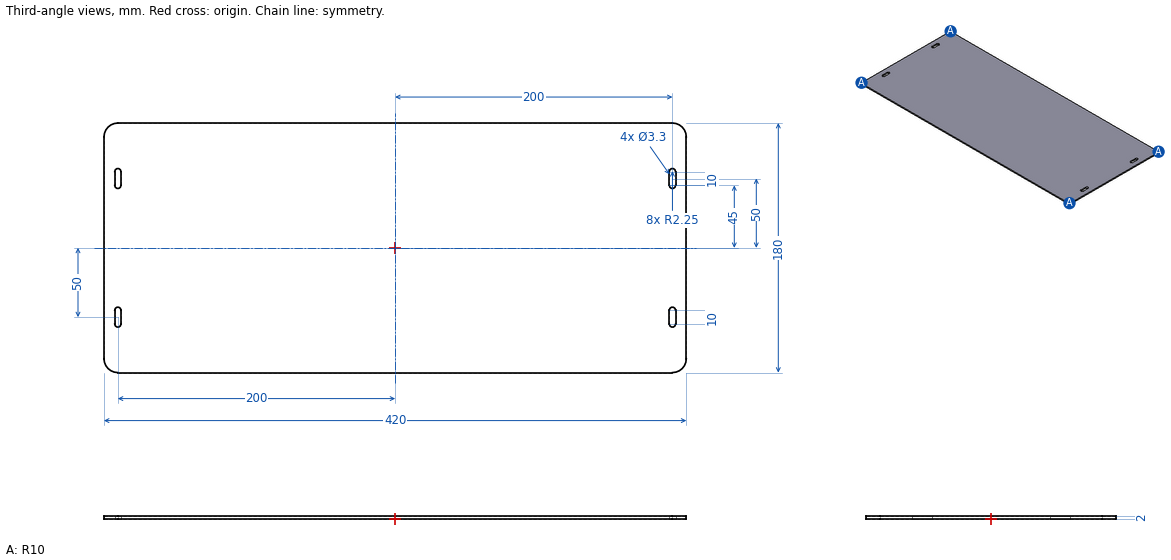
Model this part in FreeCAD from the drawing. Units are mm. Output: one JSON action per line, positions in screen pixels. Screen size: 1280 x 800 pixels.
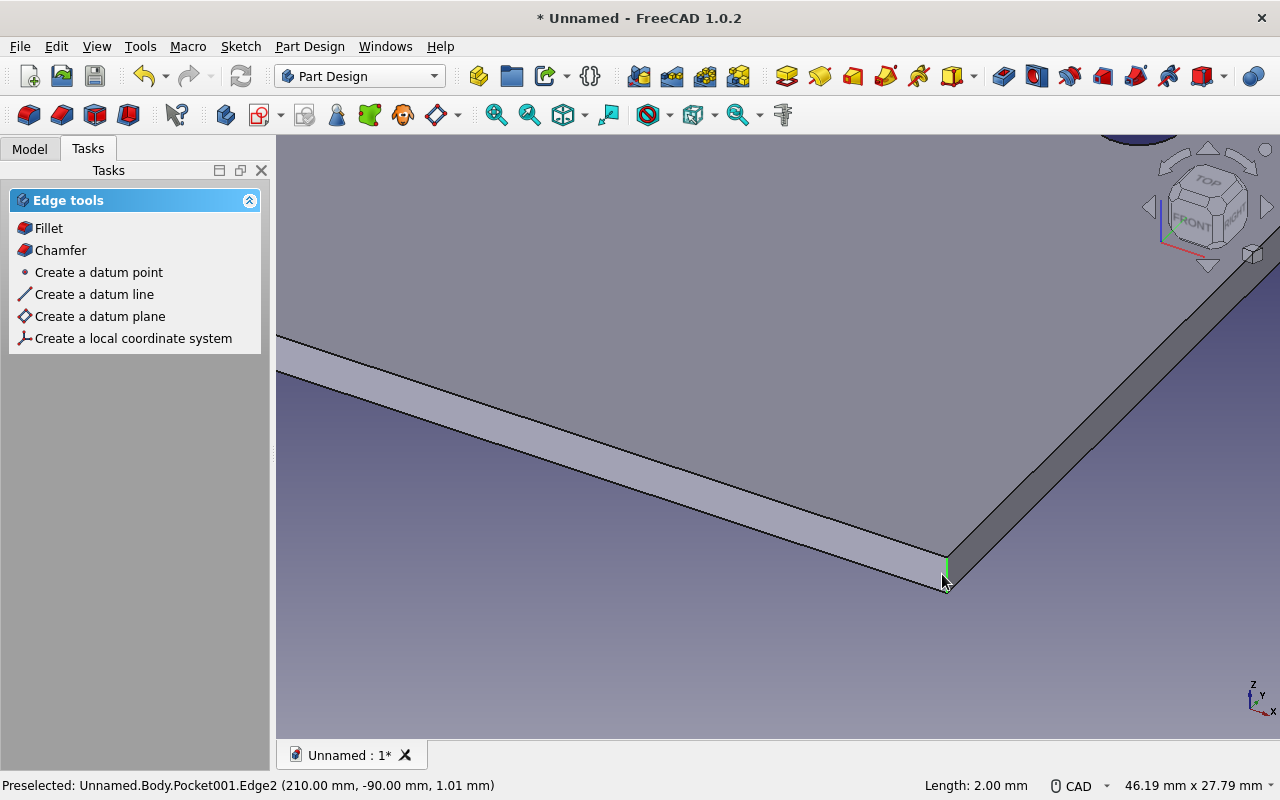
{"action": "left_click", "coordinate": [497, 116]}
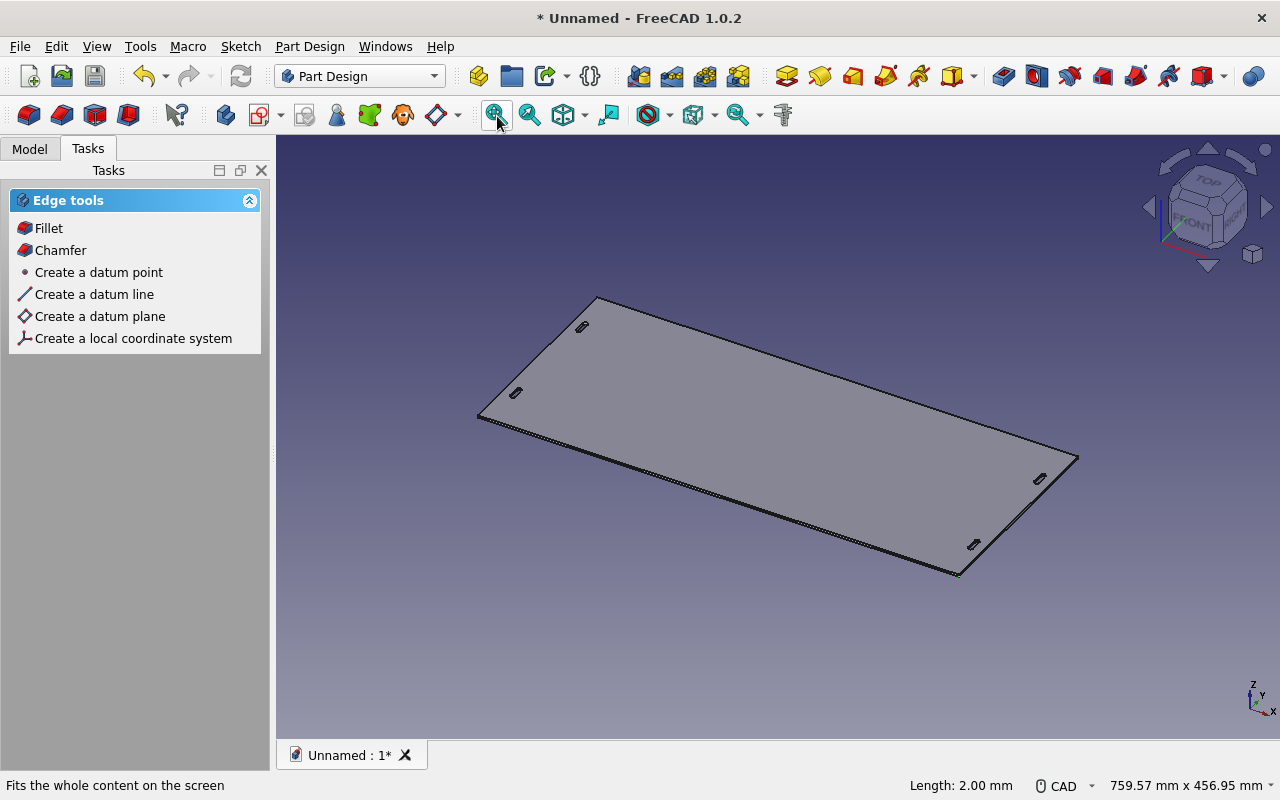
{"action": "key", "text": "0"}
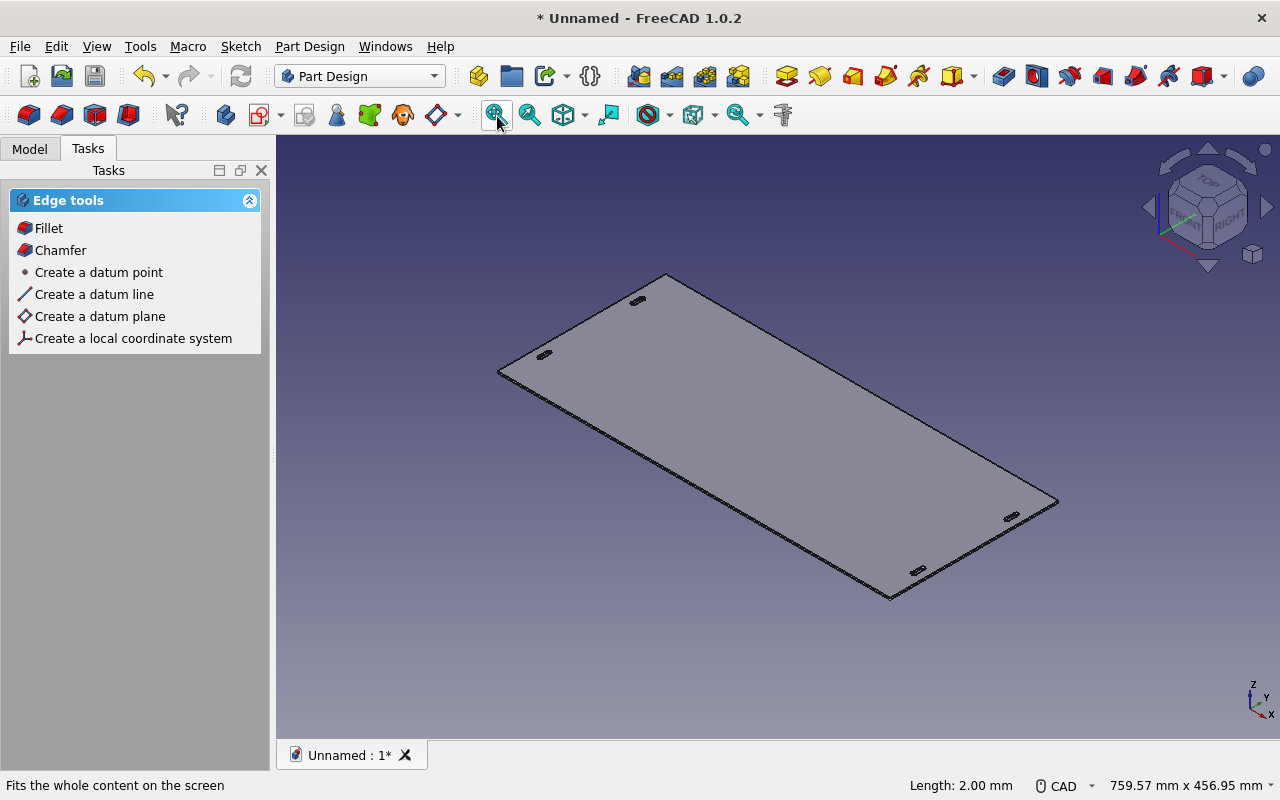
{"action": "scroll", "coordinate": [498, 371], "scroll_direction": "up", "scroll_amount": 14}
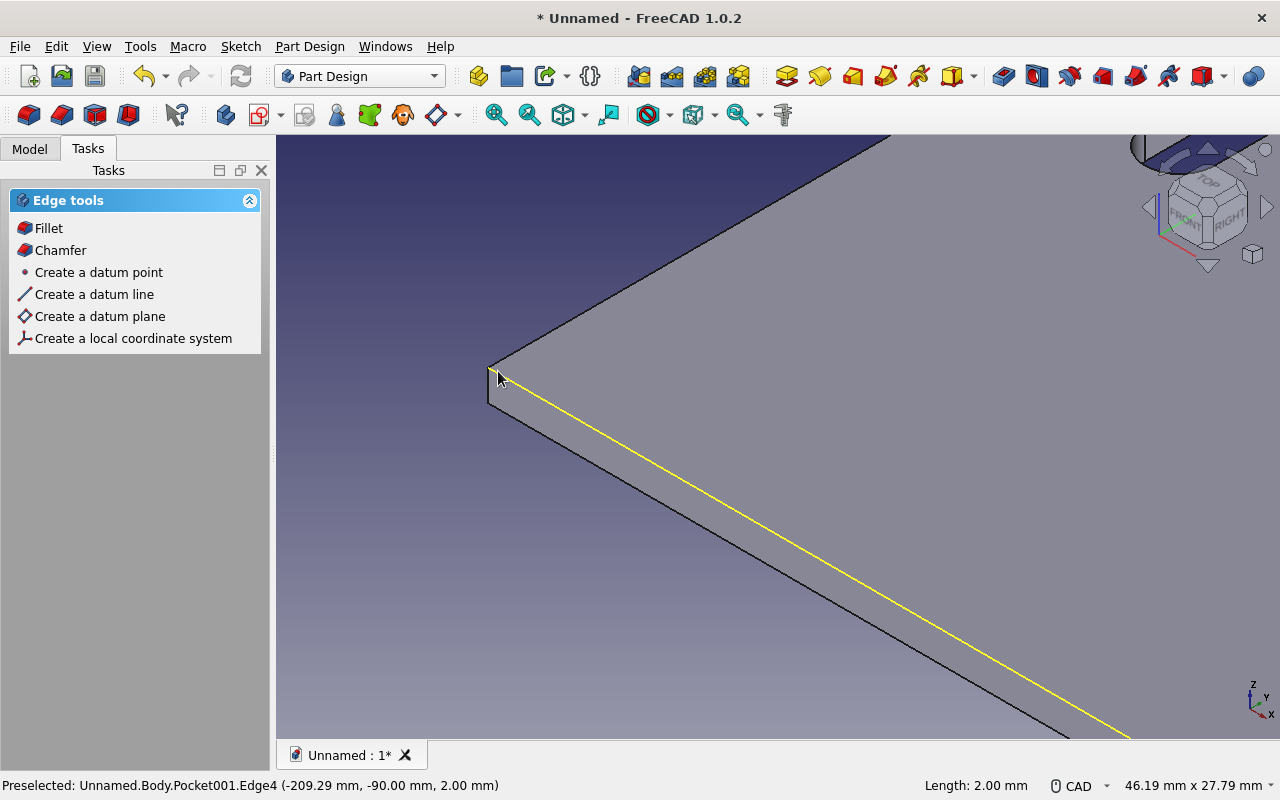
{"action": "key", "text": "v f"}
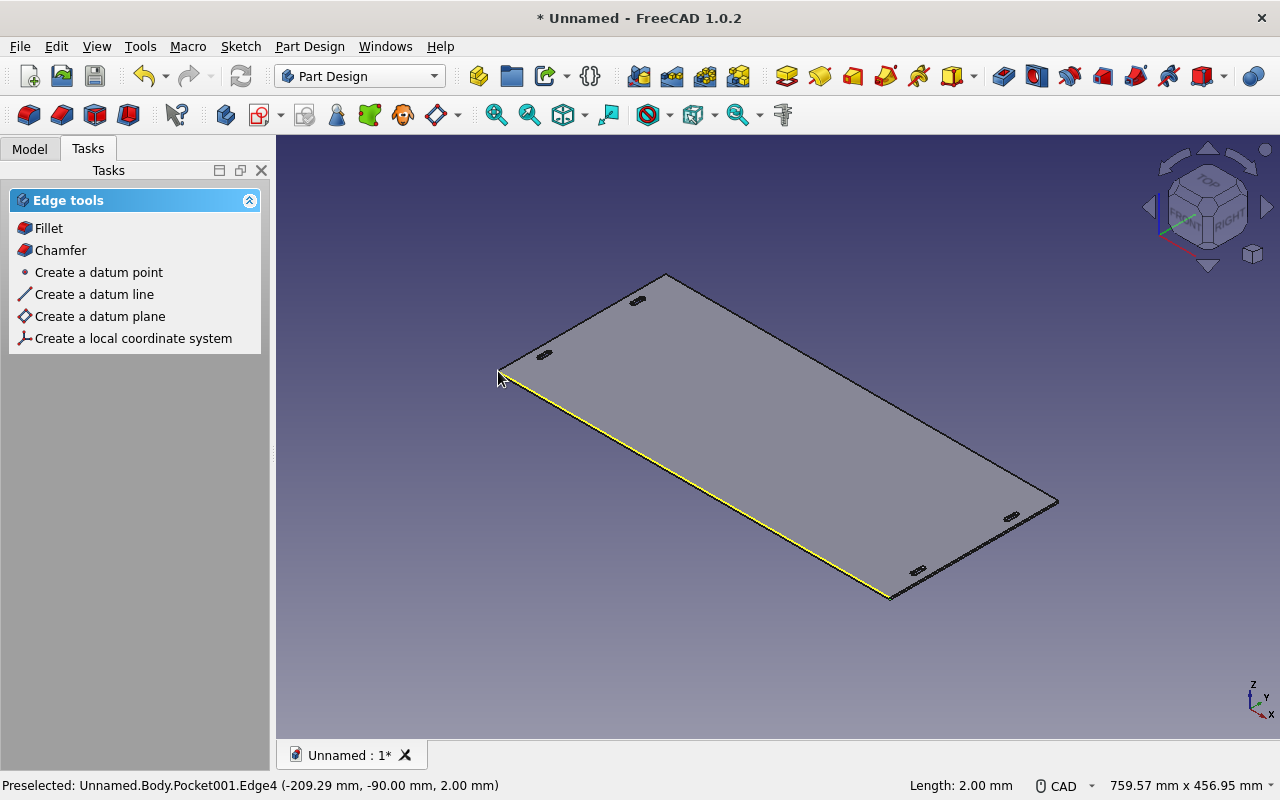
{"action": "key", "text": "2"}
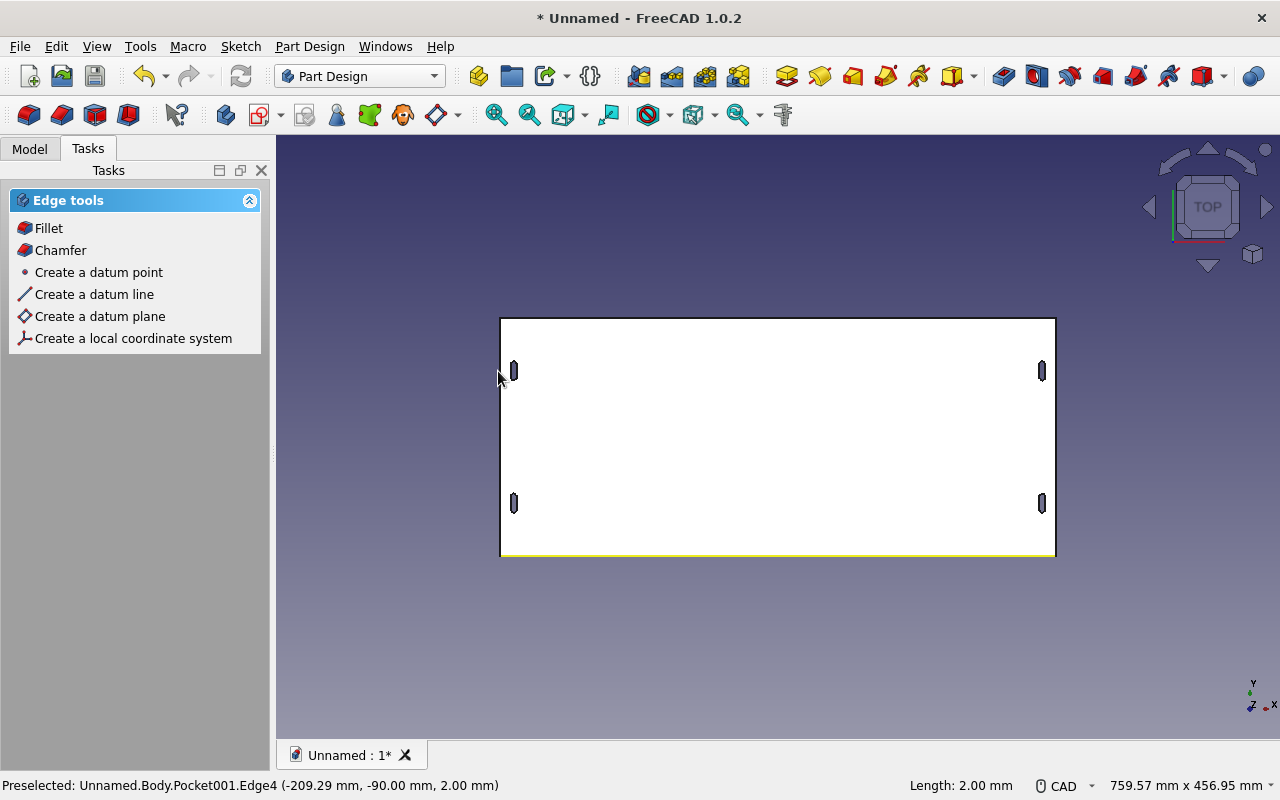
{"action": "scroll", "coordinate": [500, 555], "scroll_direction": "up", "scroll_amount": 14}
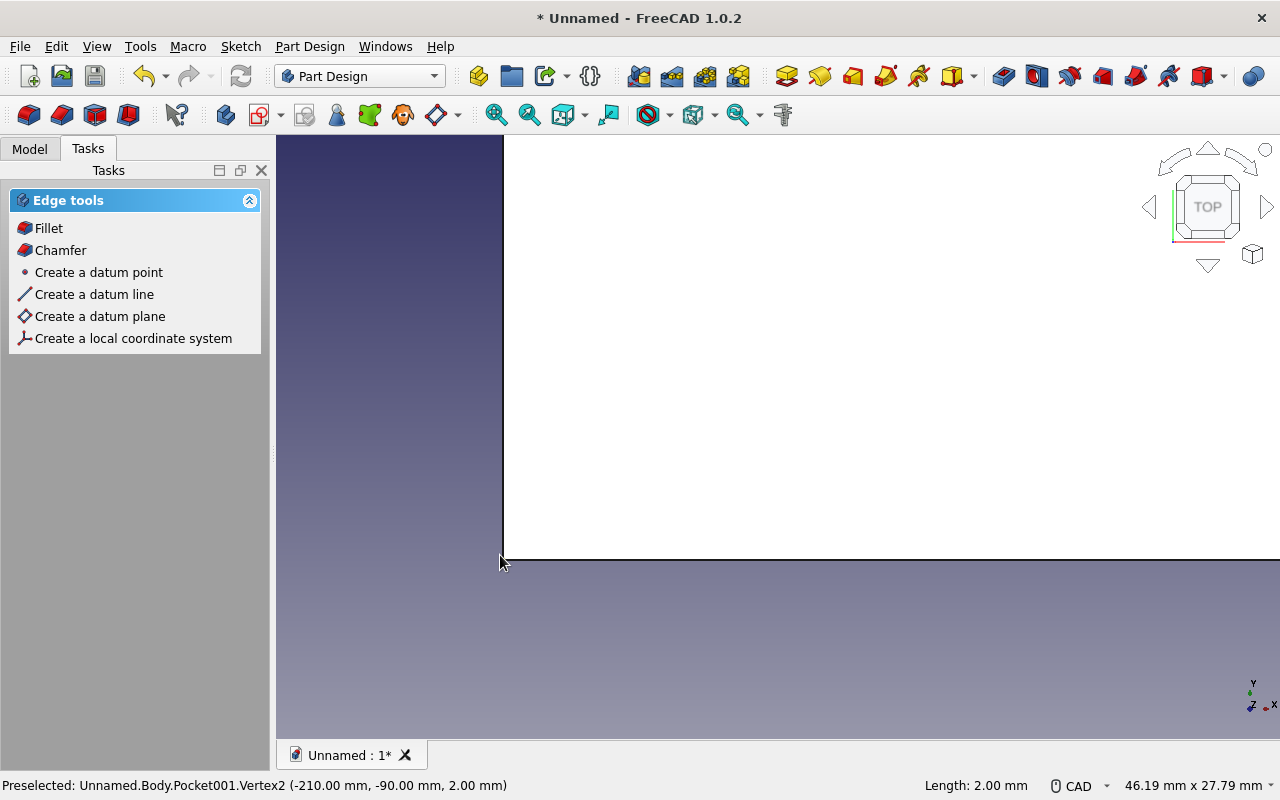
{"action": "key", "text": "v f"}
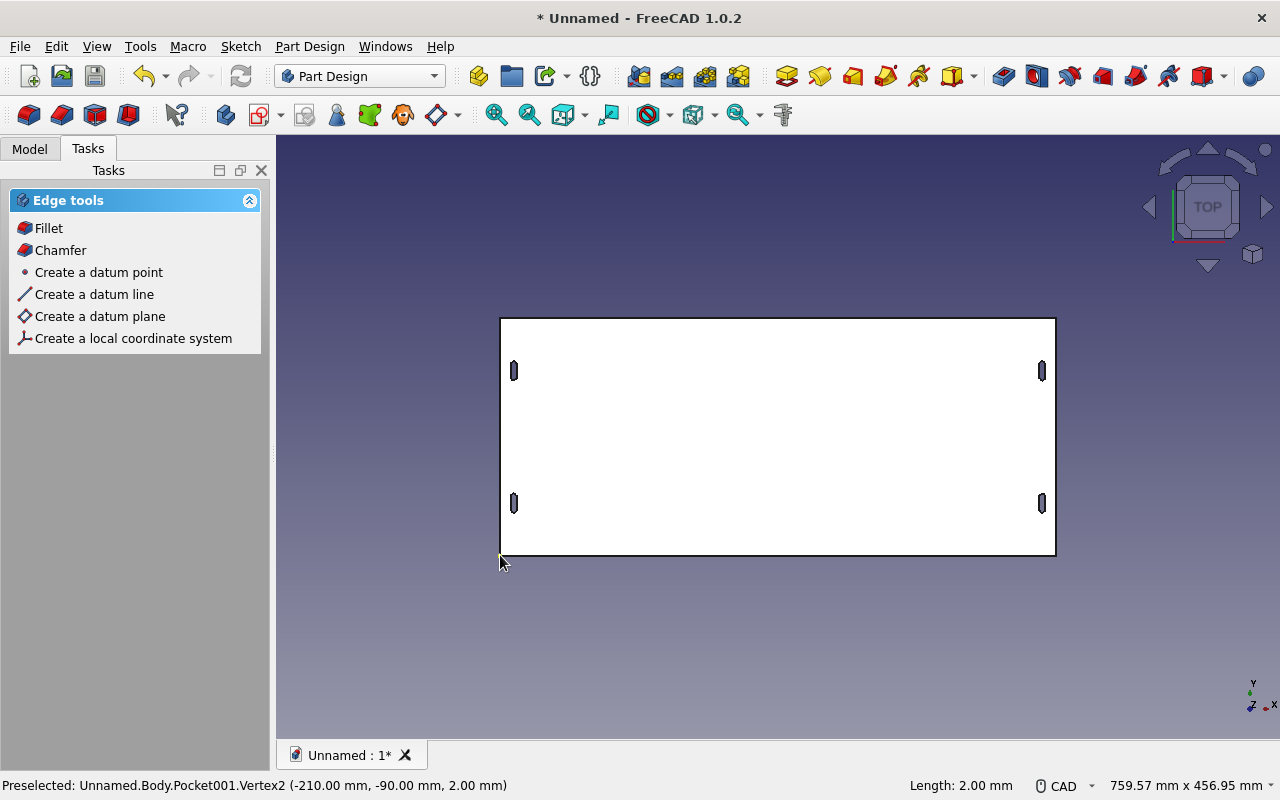
{"action": "key", "text": "1"}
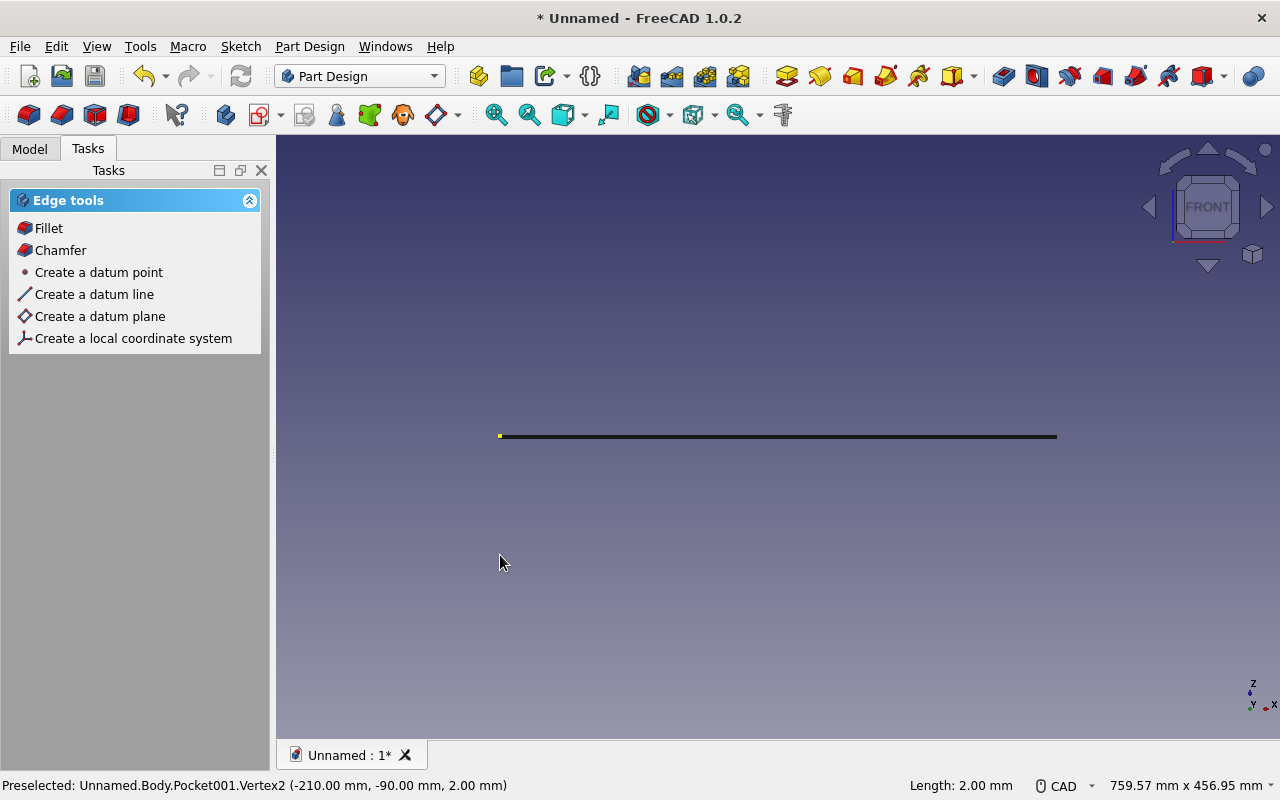
{"action": "scroll", "coordinate": [500, 436], "scroll_direction": "up", "scroll_amount": 14}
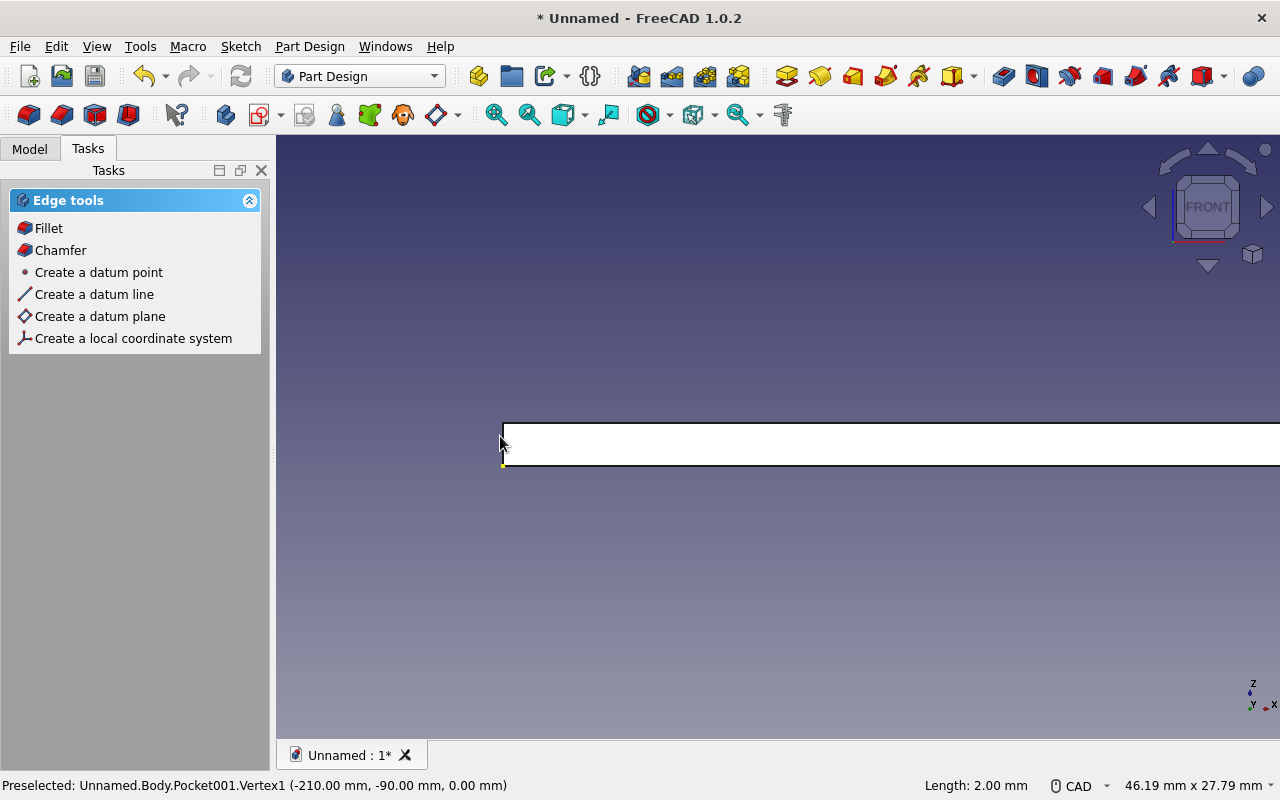
{"action": "left_click", "coordinate": [503, 444], "text": "ctrl"}